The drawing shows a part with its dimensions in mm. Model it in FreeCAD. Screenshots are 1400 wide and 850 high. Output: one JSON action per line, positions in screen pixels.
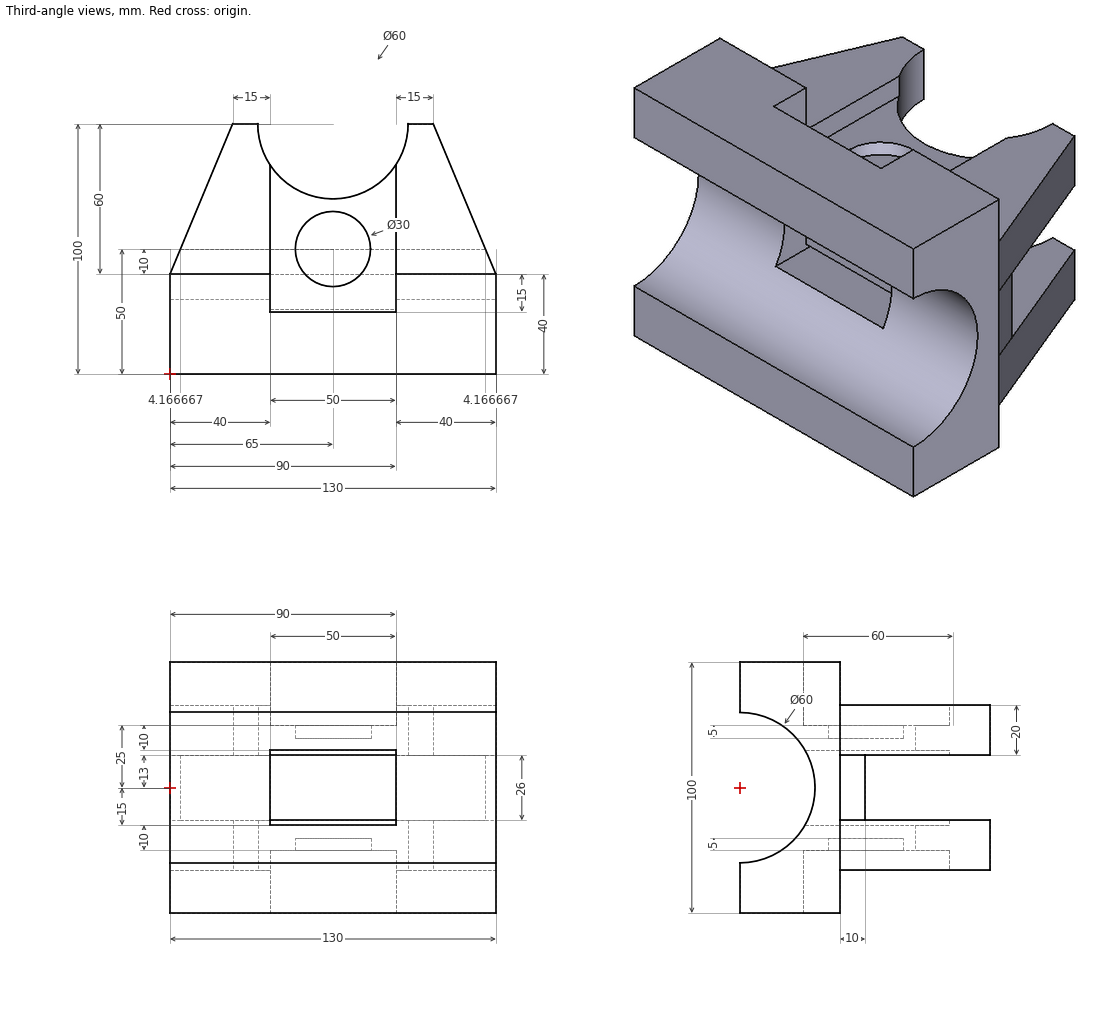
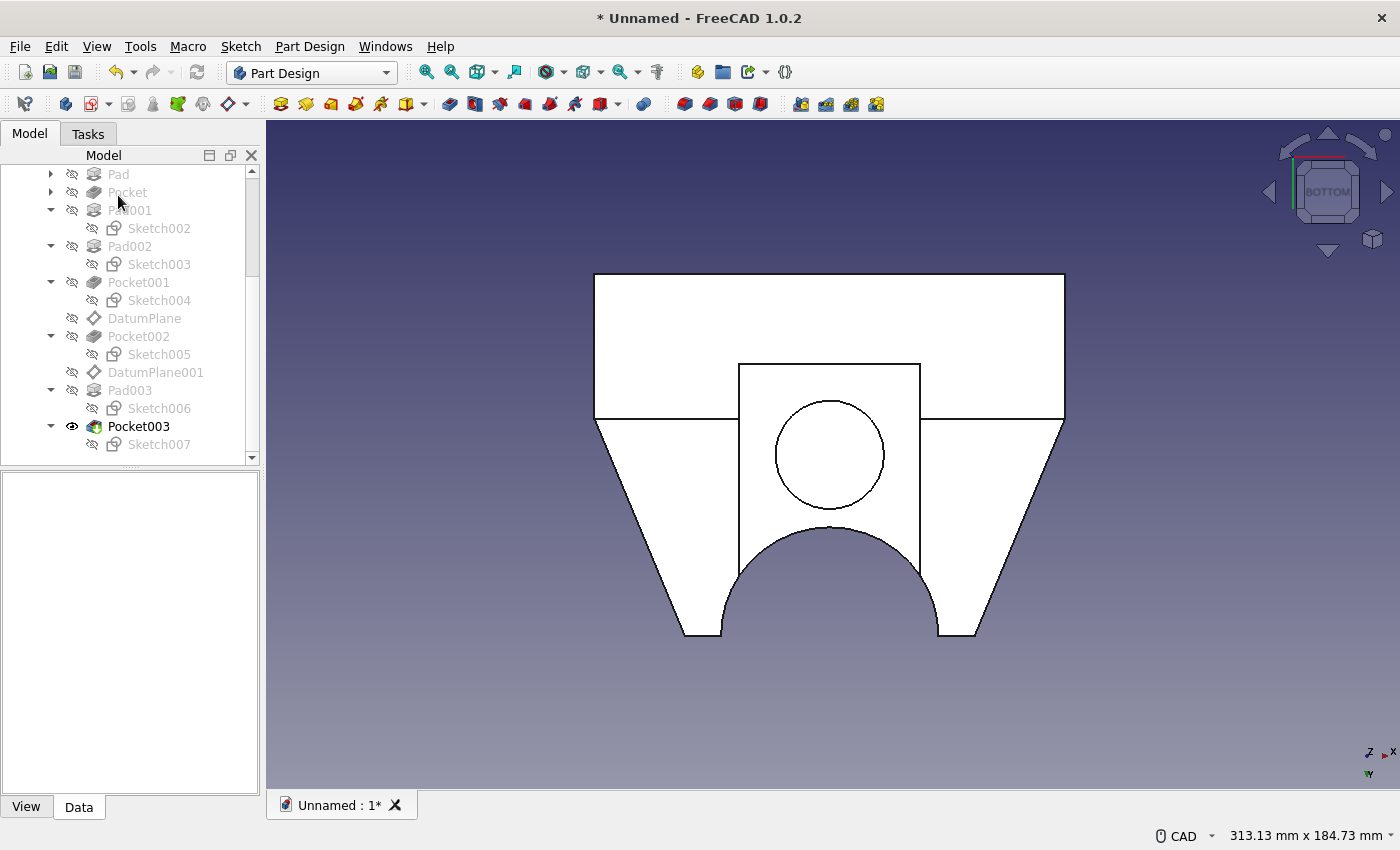
{"action": "left_click", "coordinate": [117, 174]}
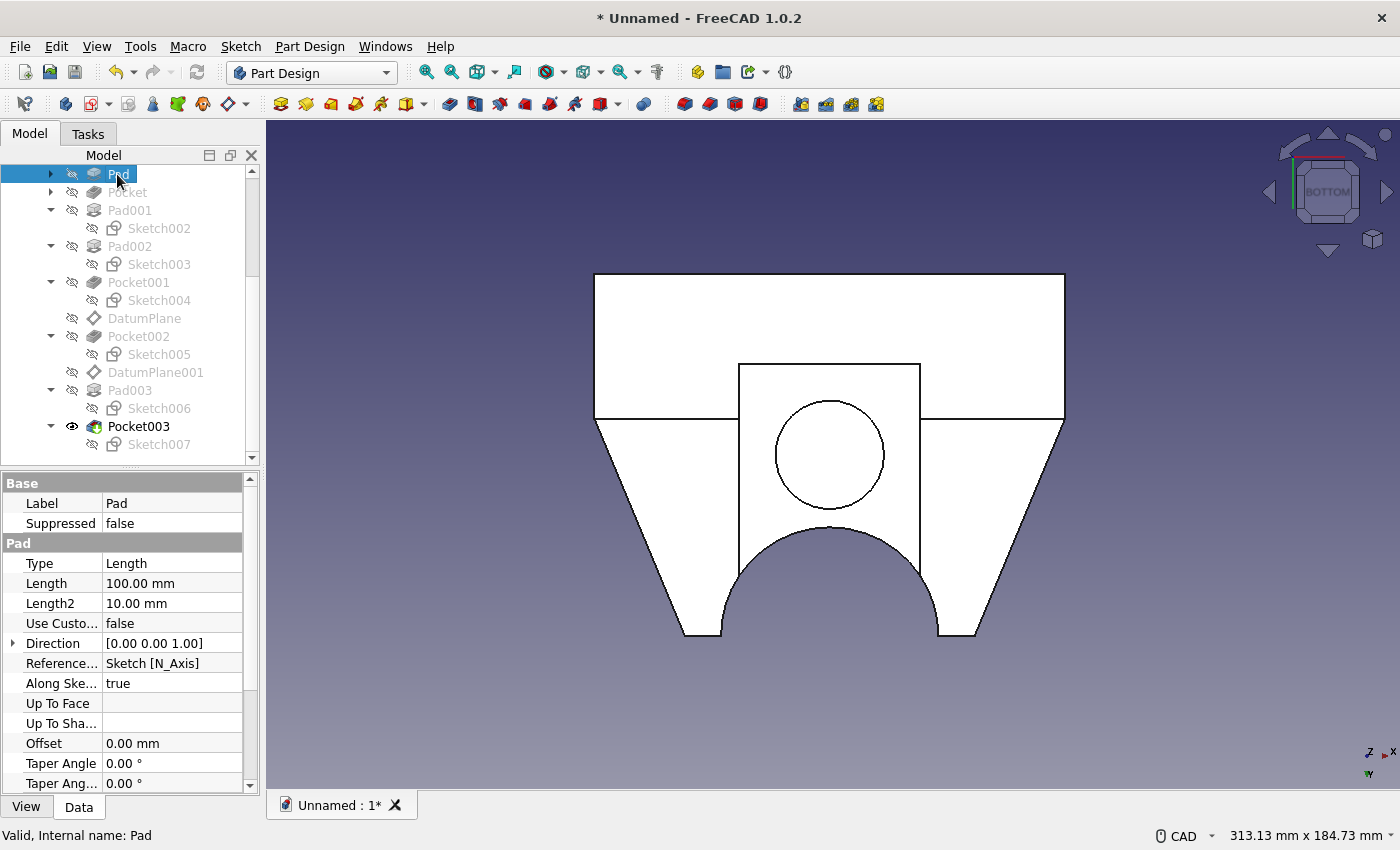
{"action": "left_click", "coordinate": [117, 390], "text": "ctrl"}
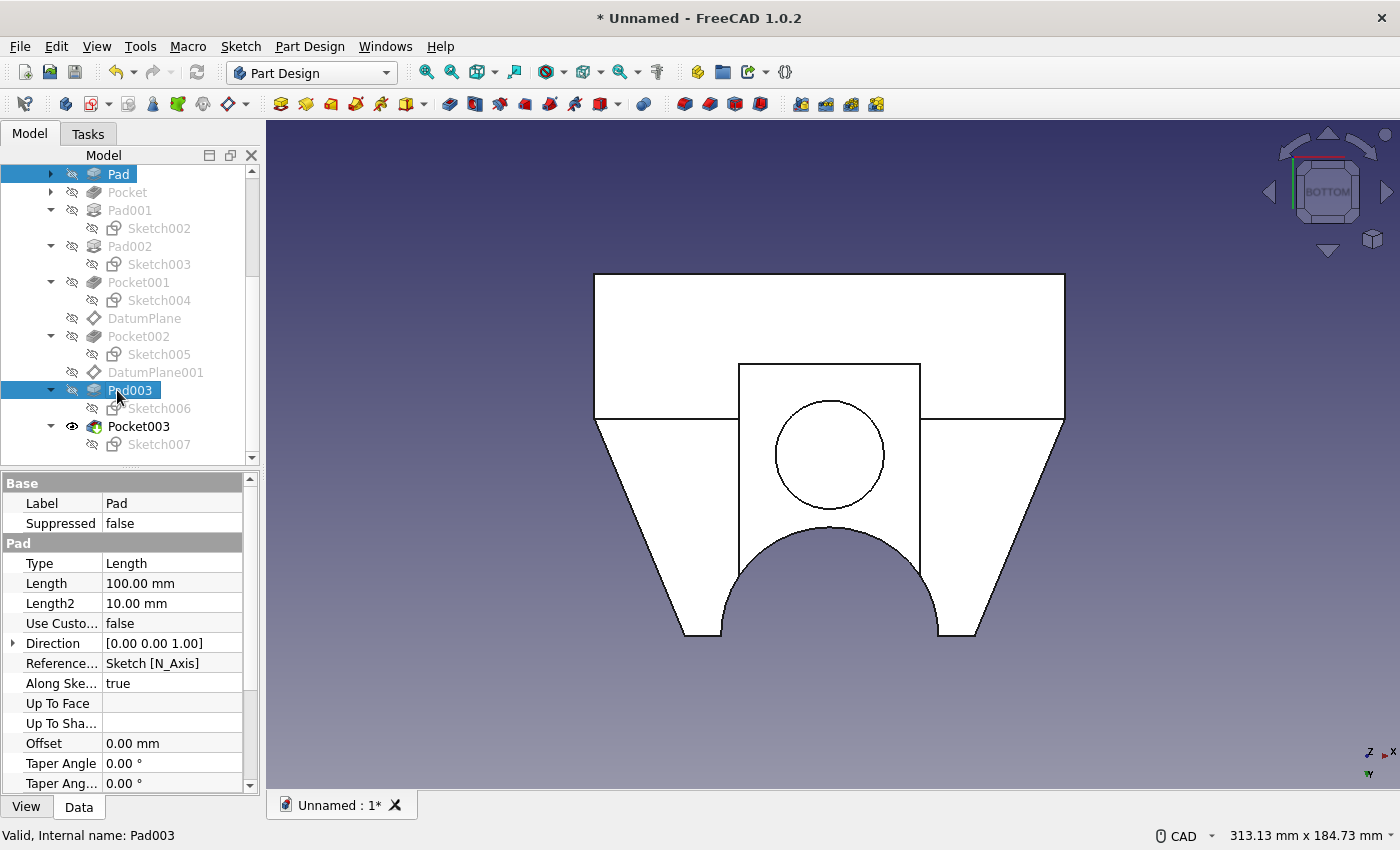
{"action": "left_click", "coordinate": [117, 426], "text": "ctrl"}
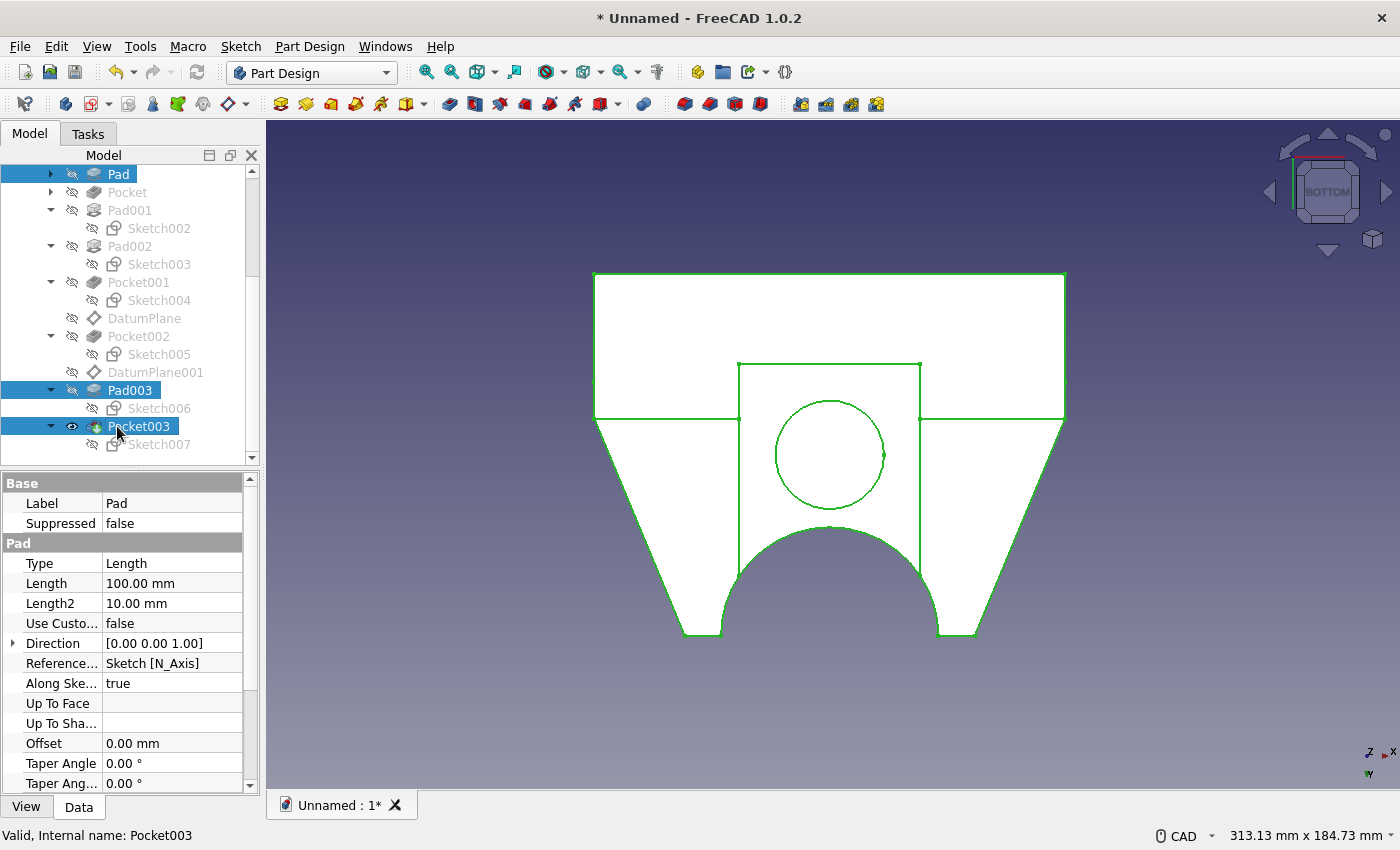
{"action": "left_click", "coordinate": [801, 104]}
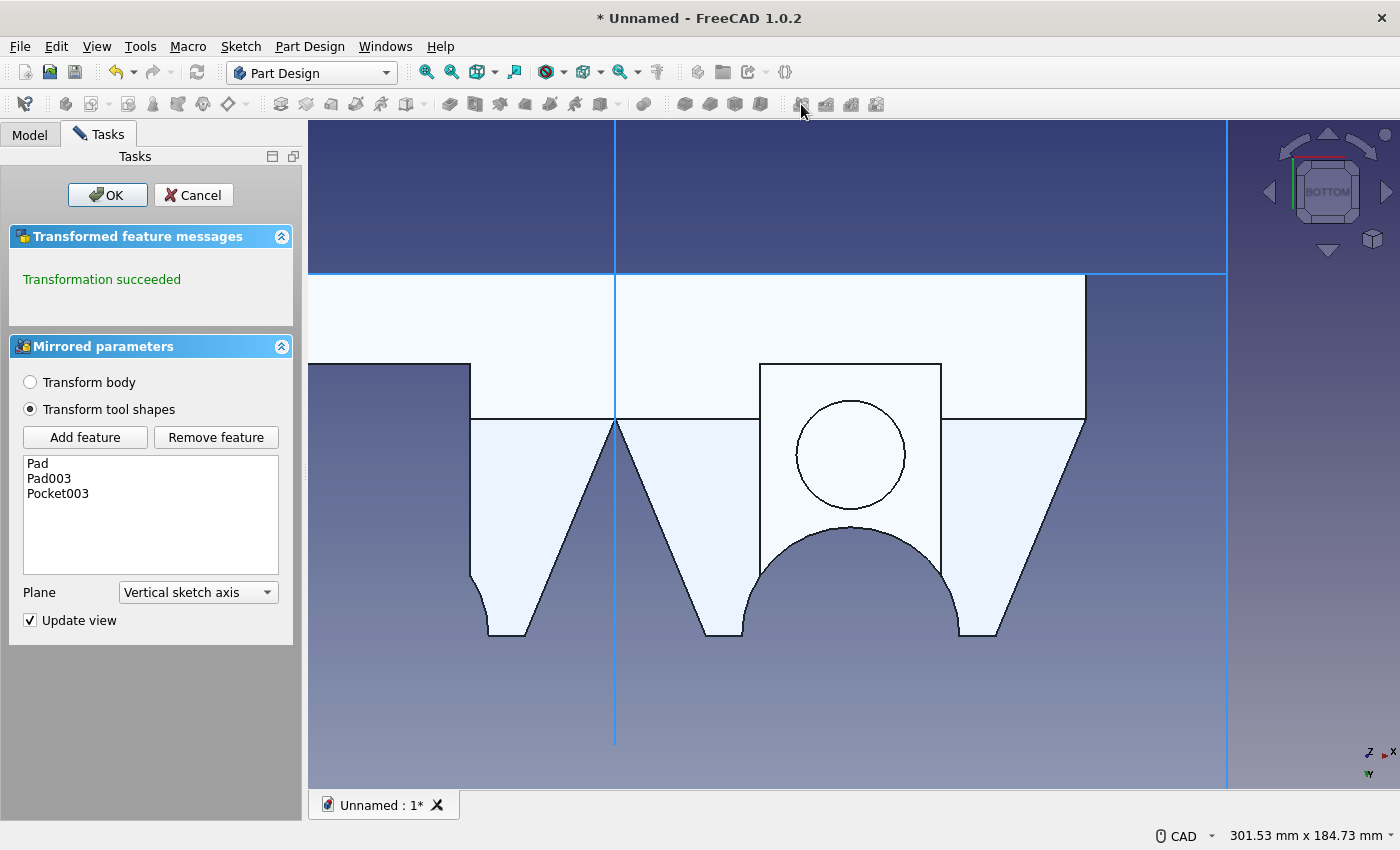
{"action": "left_click", "coordinate": [199, 592]}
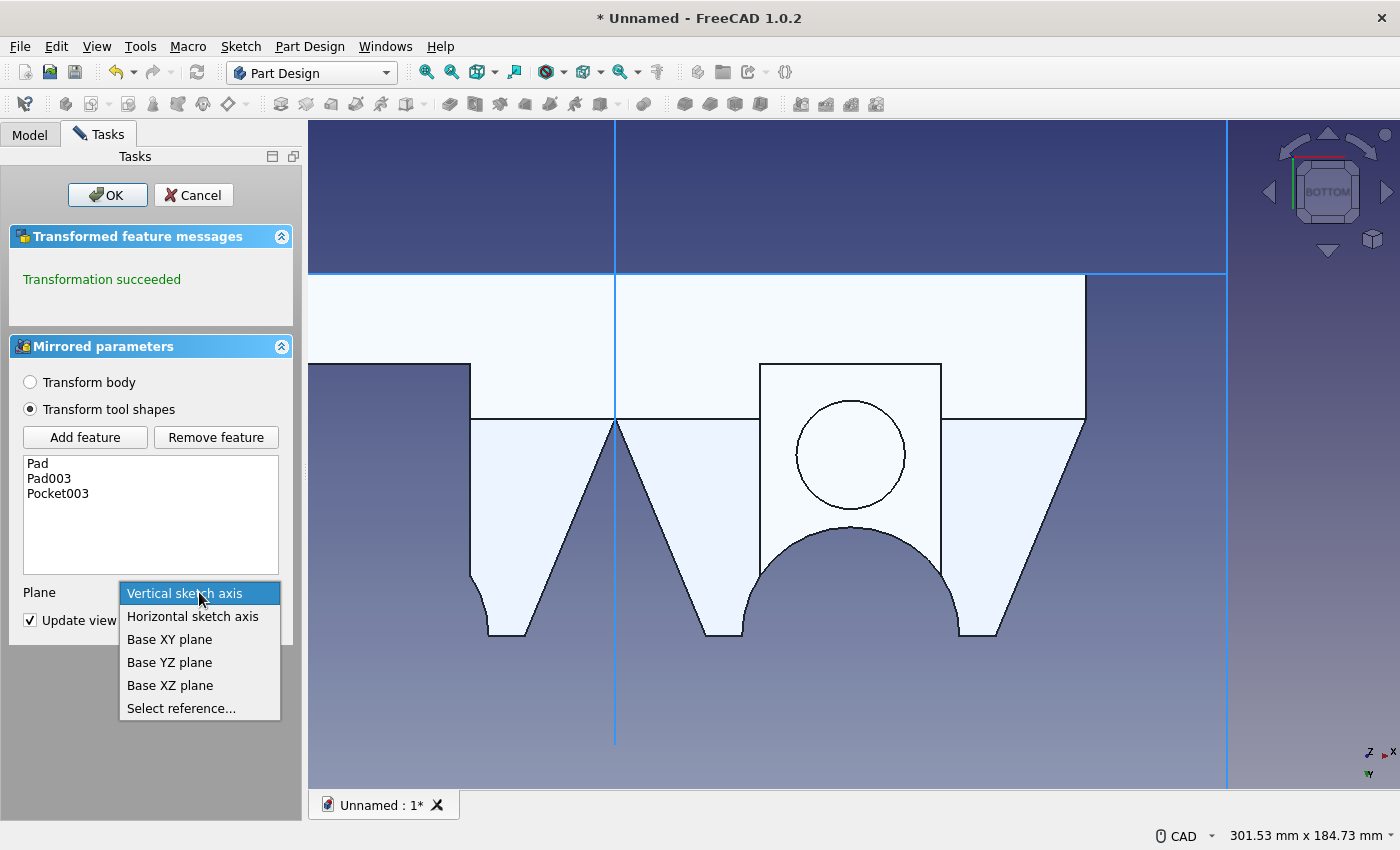
{"action": "left_click", "coordinate": [198, 640]}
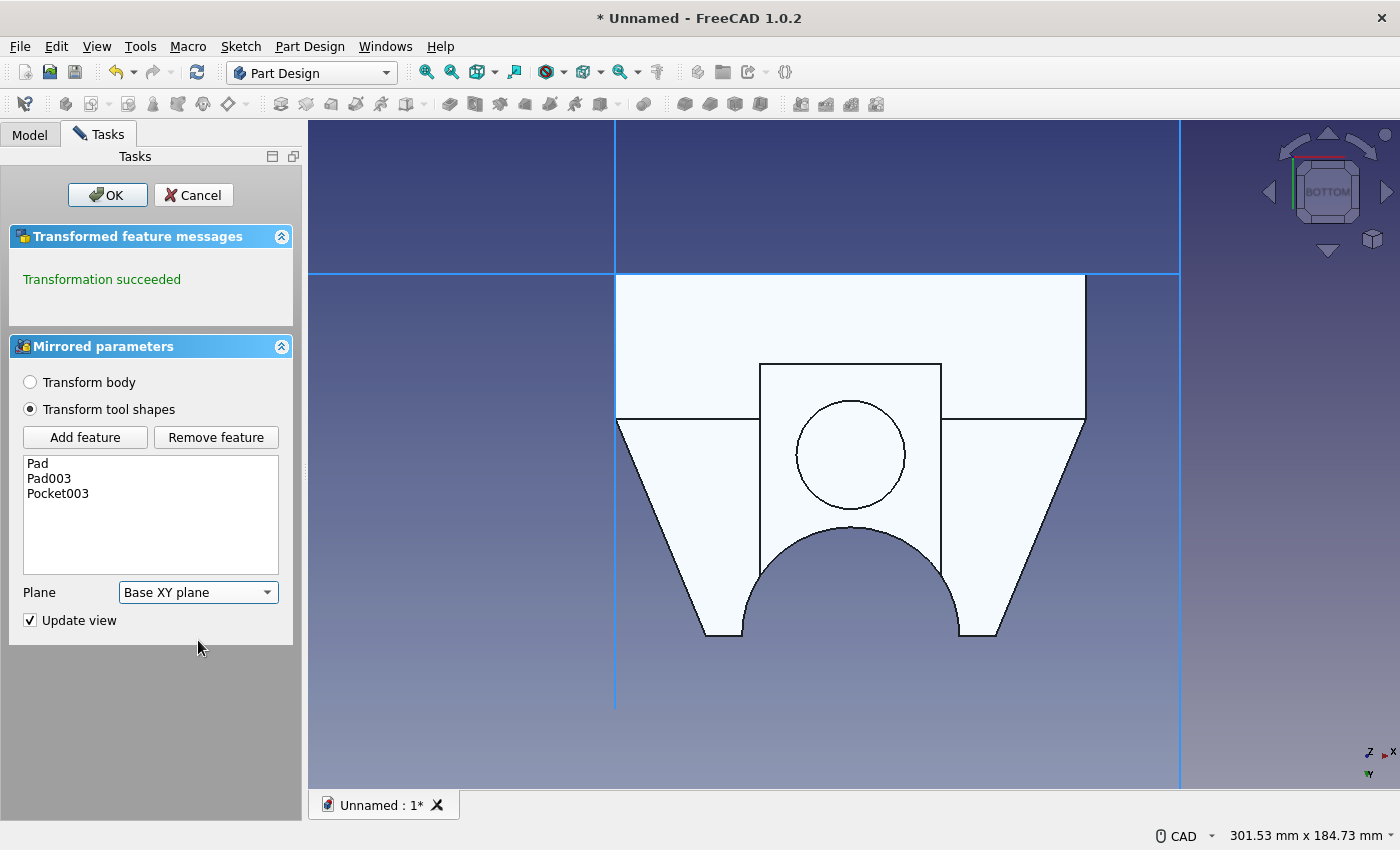
{"action": "left_click", "coordinate": [108, 195]}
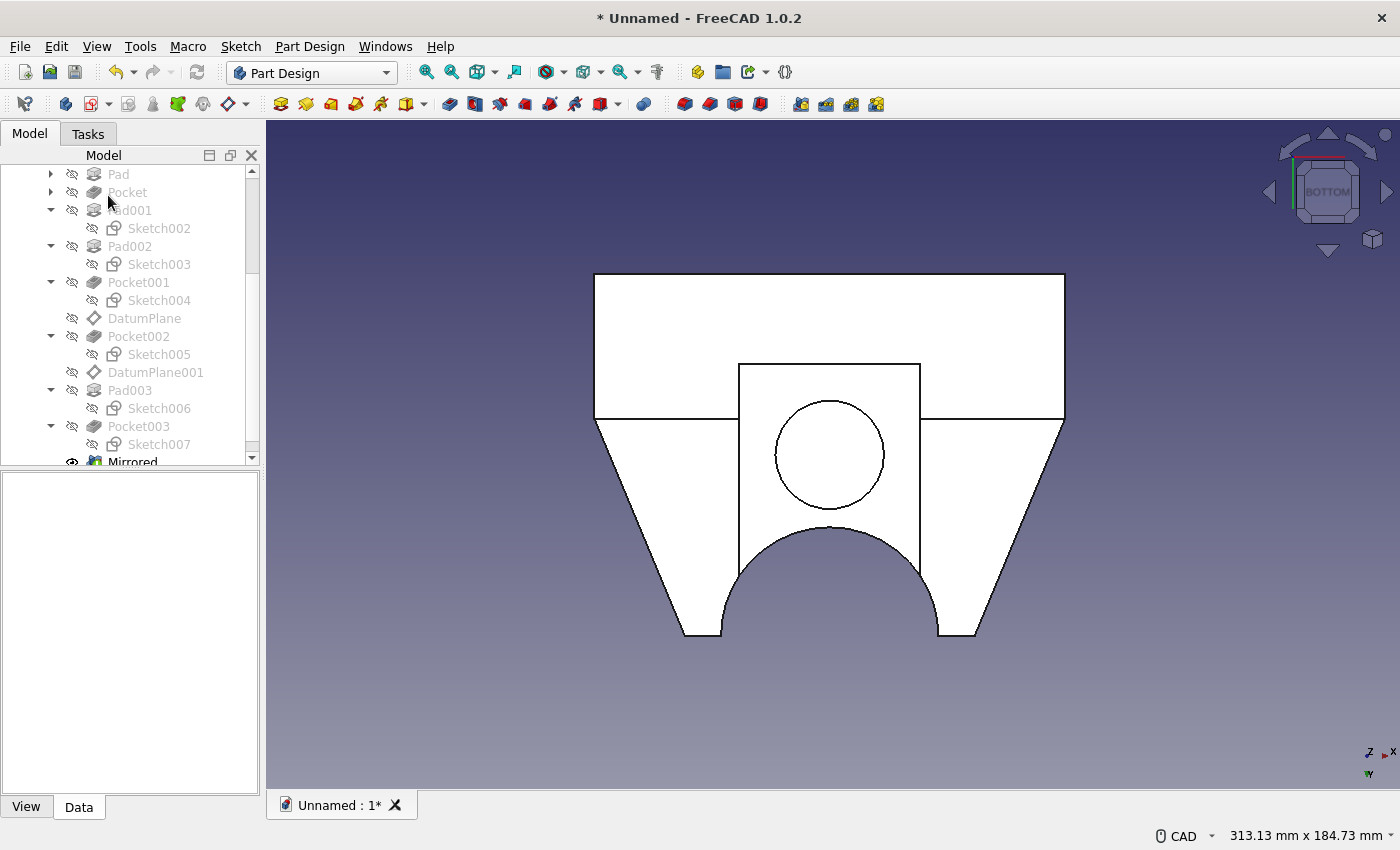
{"action": "key", "text": "4"}